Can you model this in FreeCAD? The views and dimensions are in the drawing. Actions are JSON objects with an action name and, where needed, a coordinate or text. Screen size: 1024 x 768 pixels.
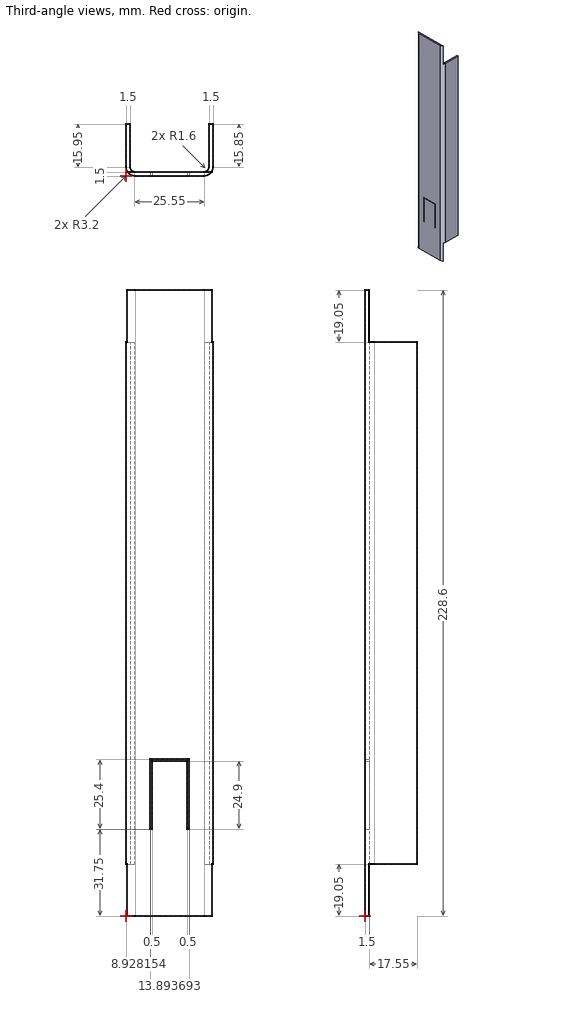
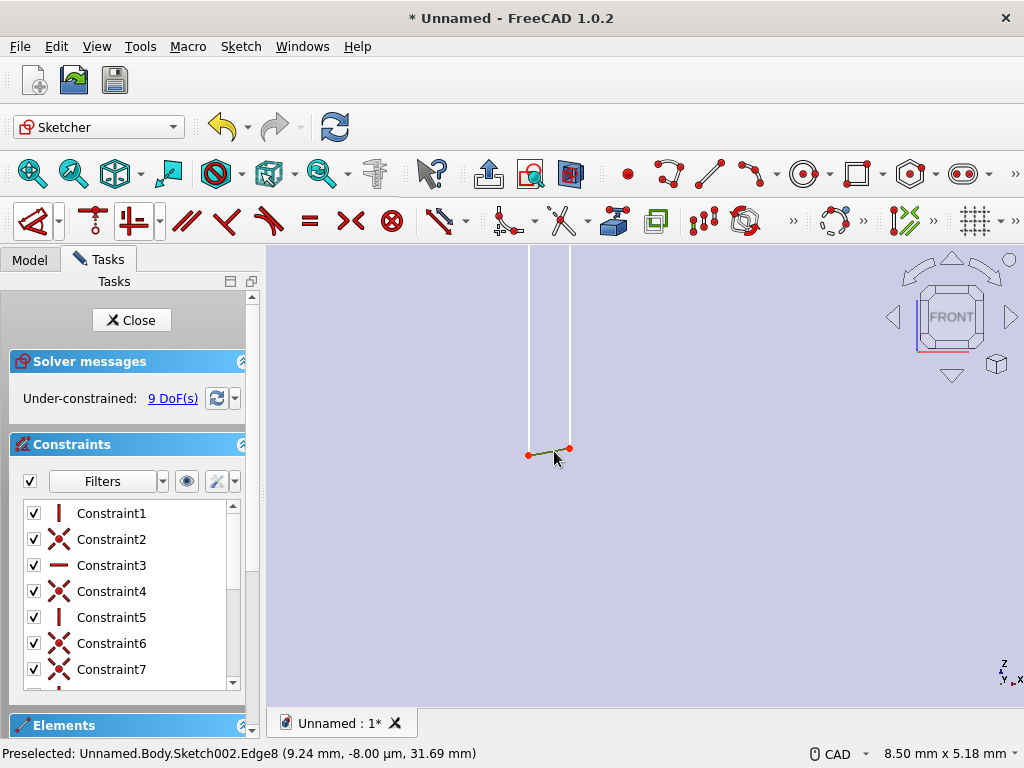
{"action": "left_click", "coordinate": [160, 222]}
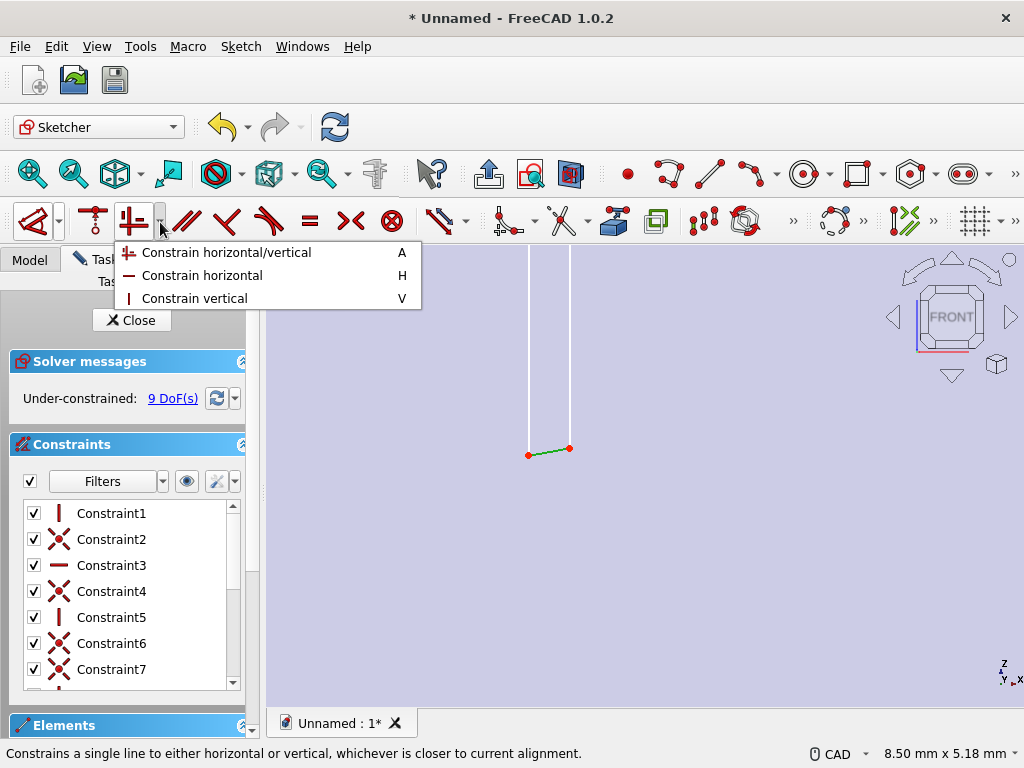
{"action": "left_click", "coordinate": [268, 276]}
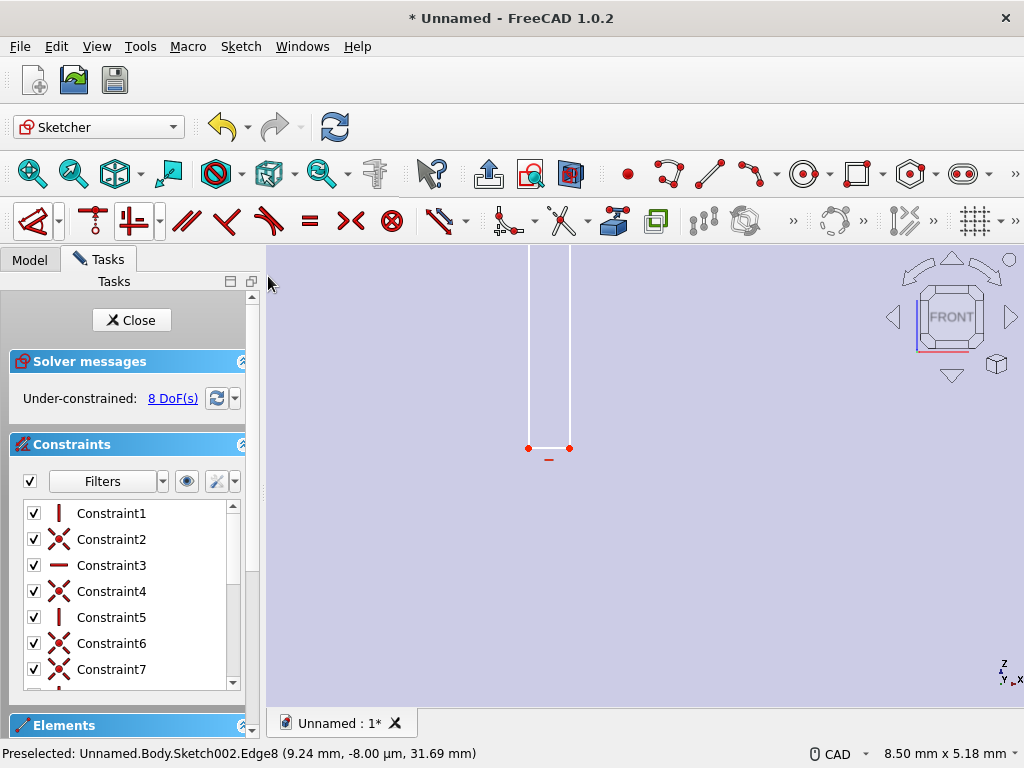
{"action": "scroll", "coordinate": [565, 460], "scroll_direction": "down", "scroll_amount": 14}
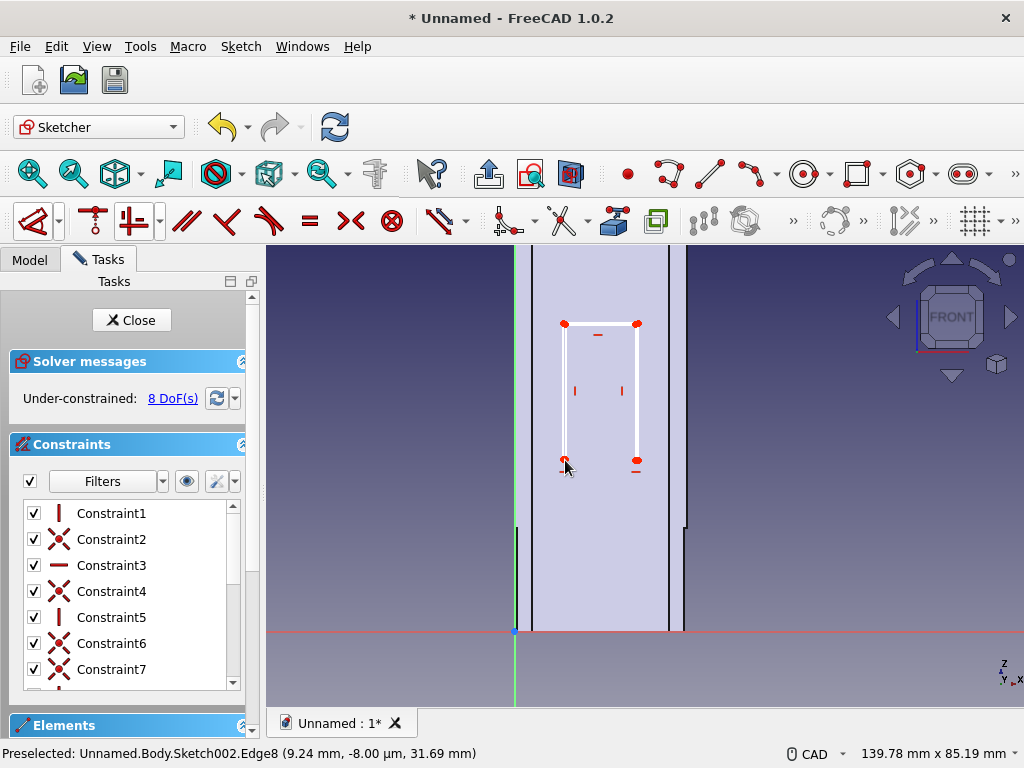
{"action": "scroll", "coordinate": [637, 460], "scroll_direction": "up", "scroll_amount": 14}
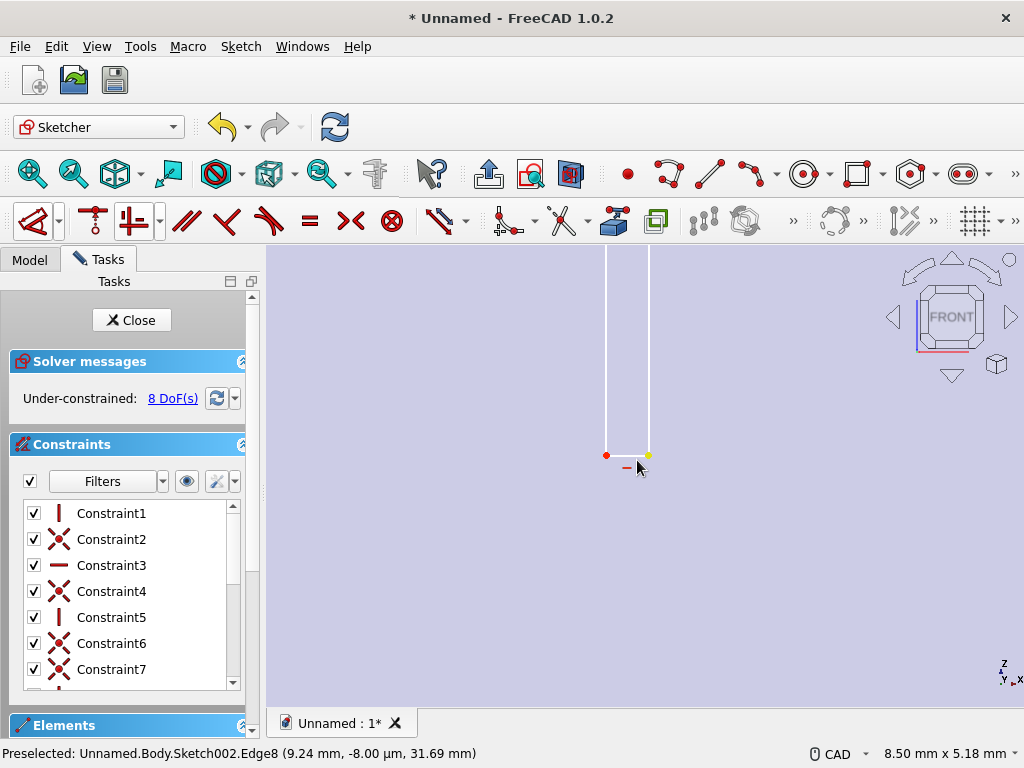
{"action": "left_click", "coordinate": [636, 456]}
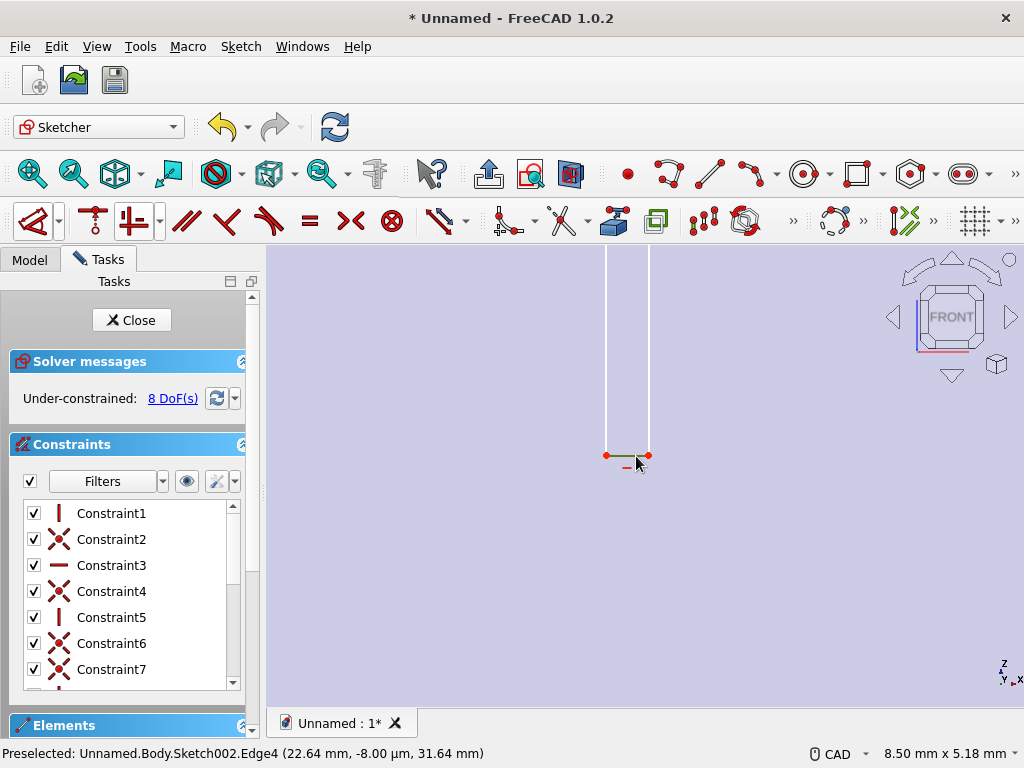
{"action": "left_click", "coordinate": [58, 222]}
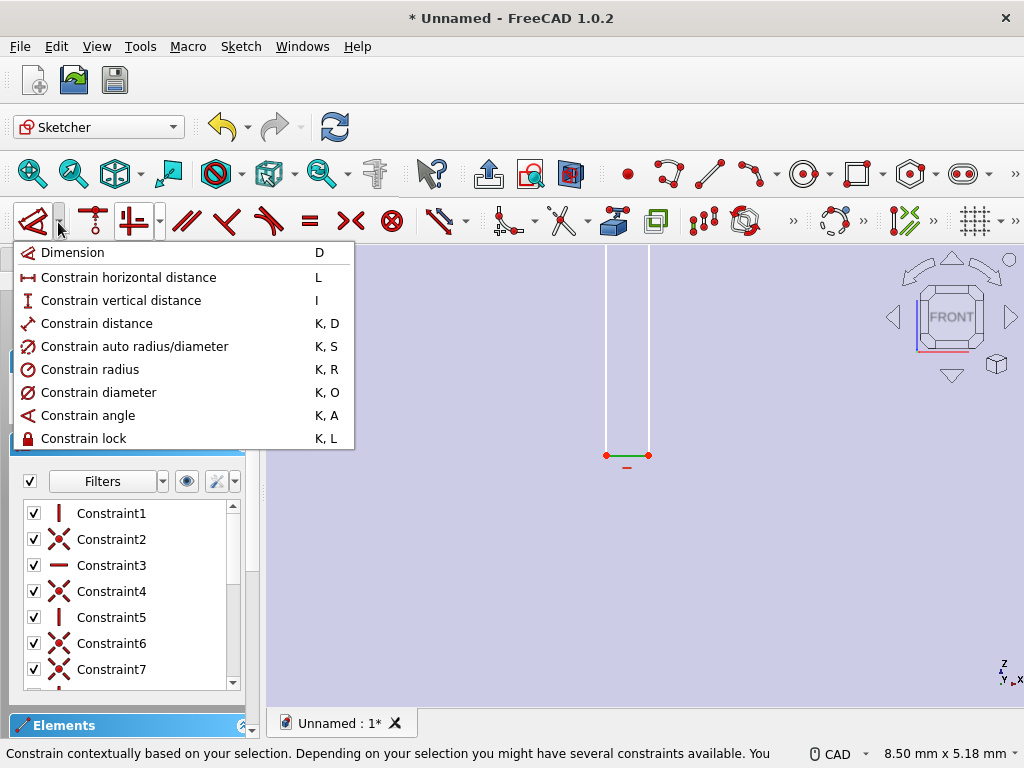
{"action": "left_click", "coordinate": [184, 278]}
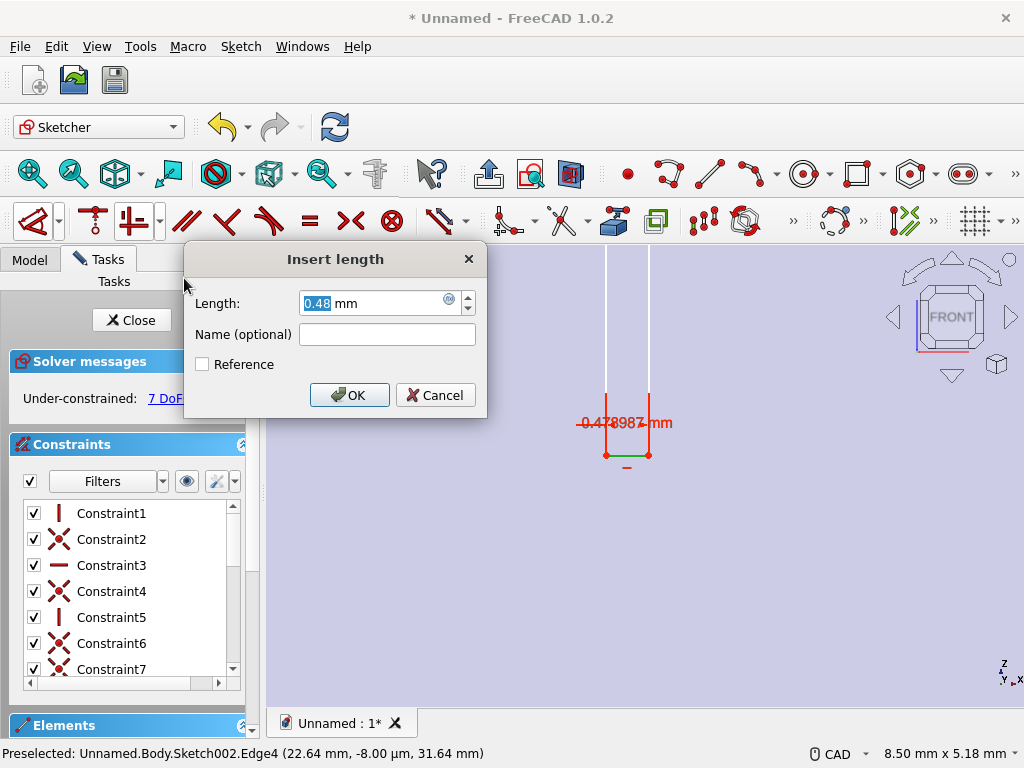
{"action": "type", "text": "0.5"}
{"action": "key", "text": "Return"}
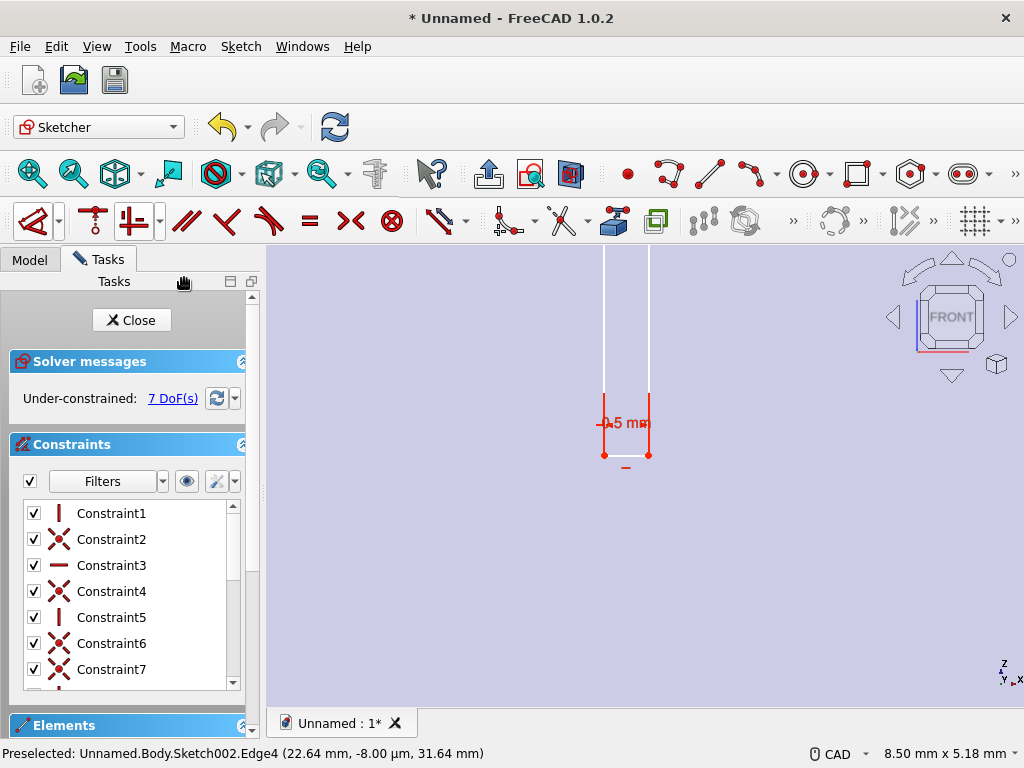
{"action": "scroll", "coordinate": [637, 460], "scroll_direction": "down", "scroll_amount": 14}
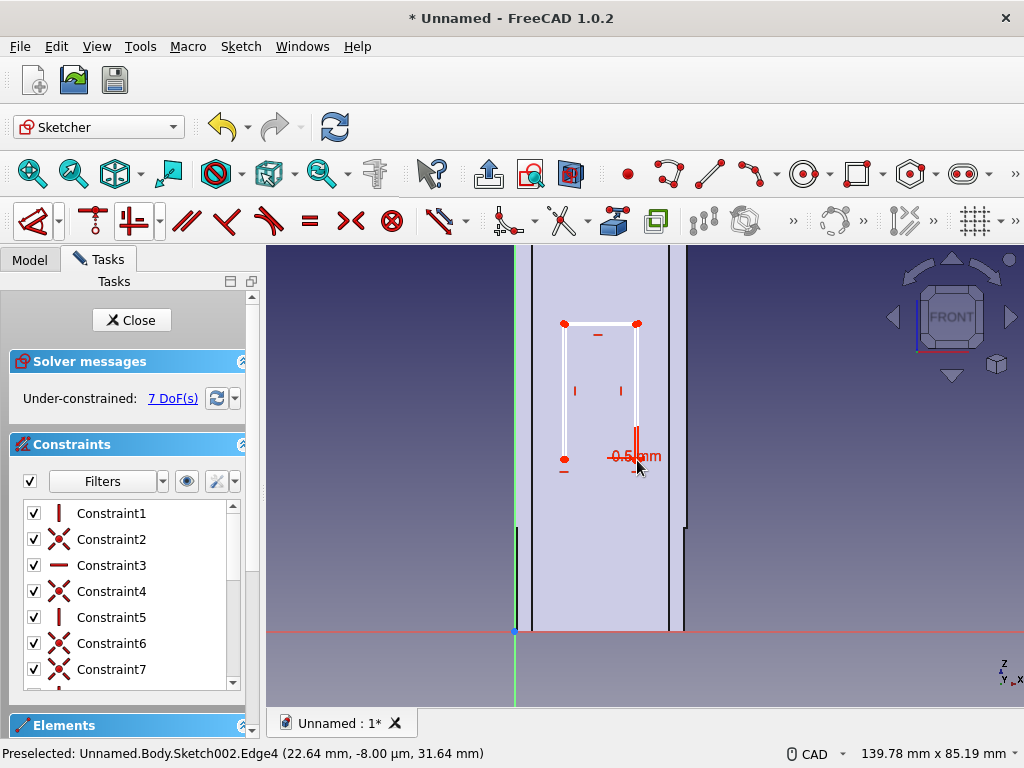
{"action": "scroll", "coordinate": [565, 460], "scroll_direction": "up", "scroll_amount": 14}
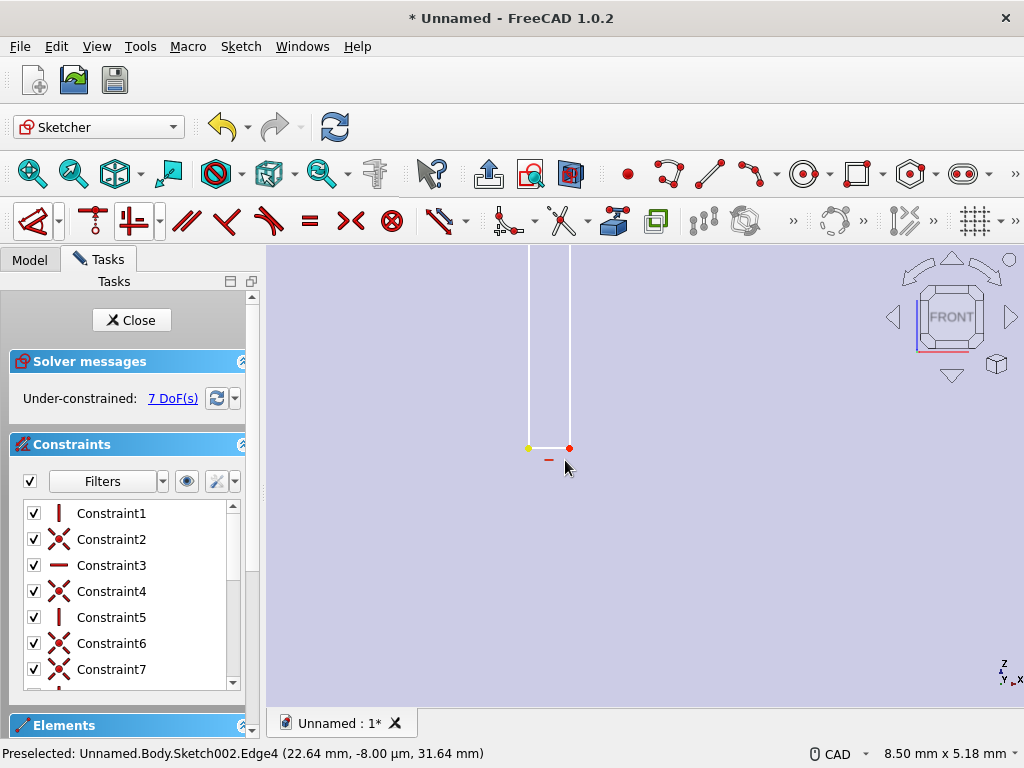
{"action": "left_click", "coordinate": [558, 448]}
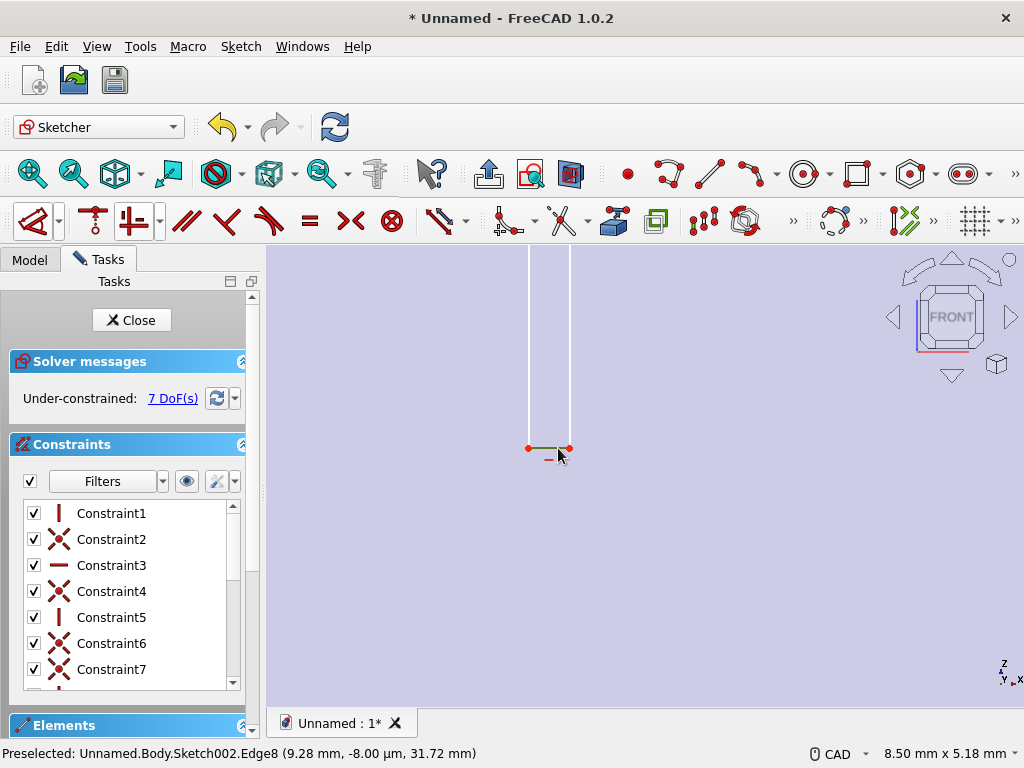
{"action": "key", "text": "l"}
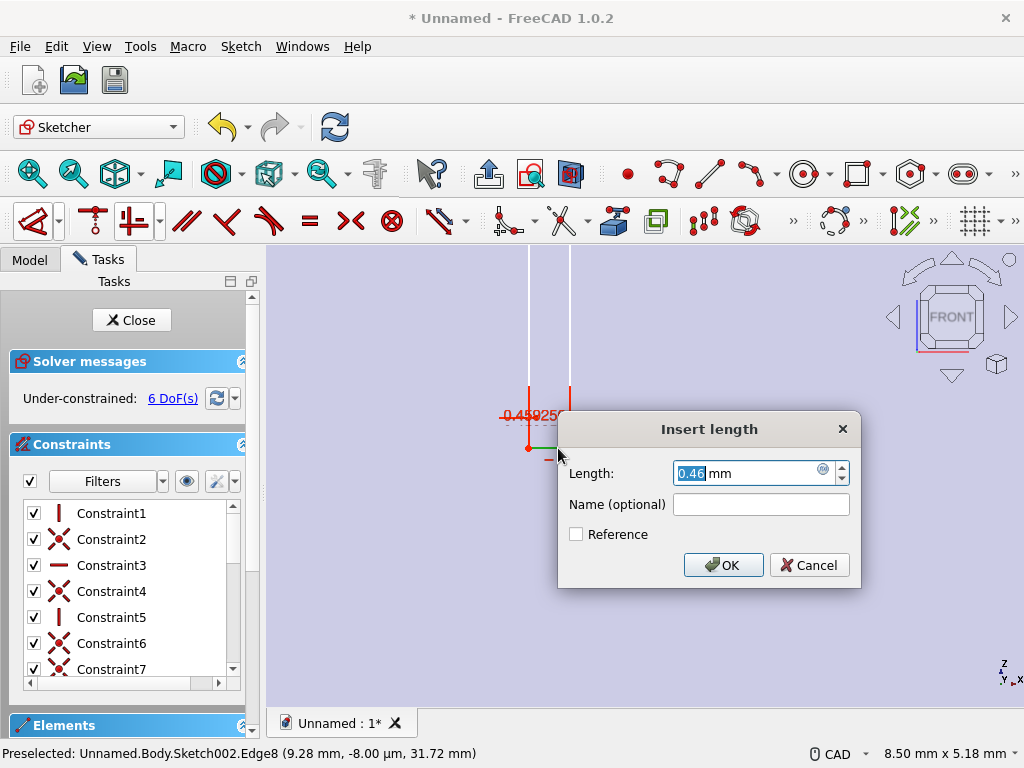
{"action": "type", "text": "0.5"}
{"action": "key", "text": "Return"}